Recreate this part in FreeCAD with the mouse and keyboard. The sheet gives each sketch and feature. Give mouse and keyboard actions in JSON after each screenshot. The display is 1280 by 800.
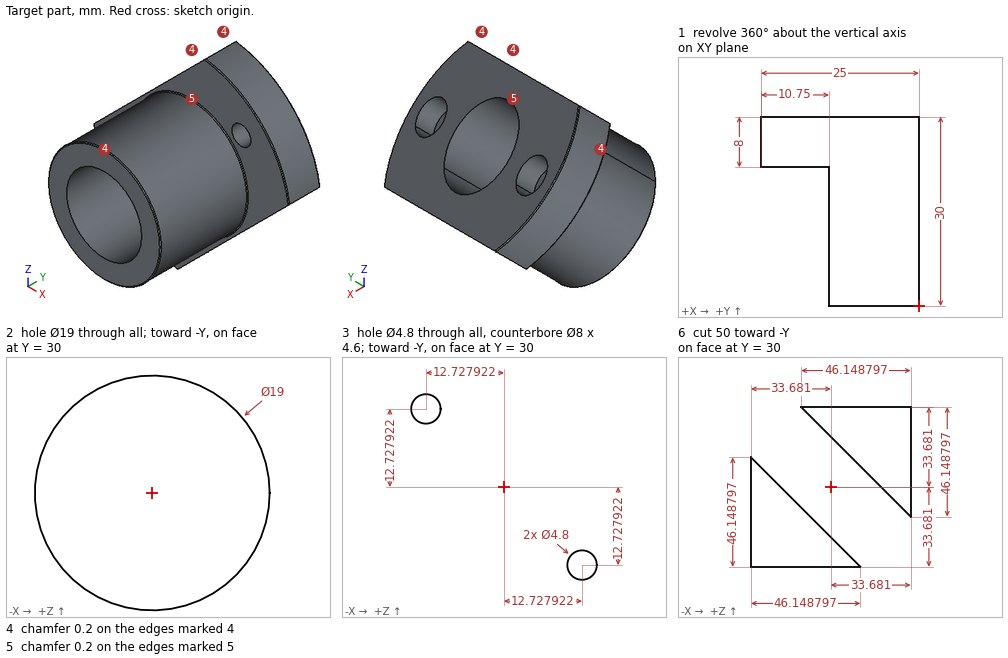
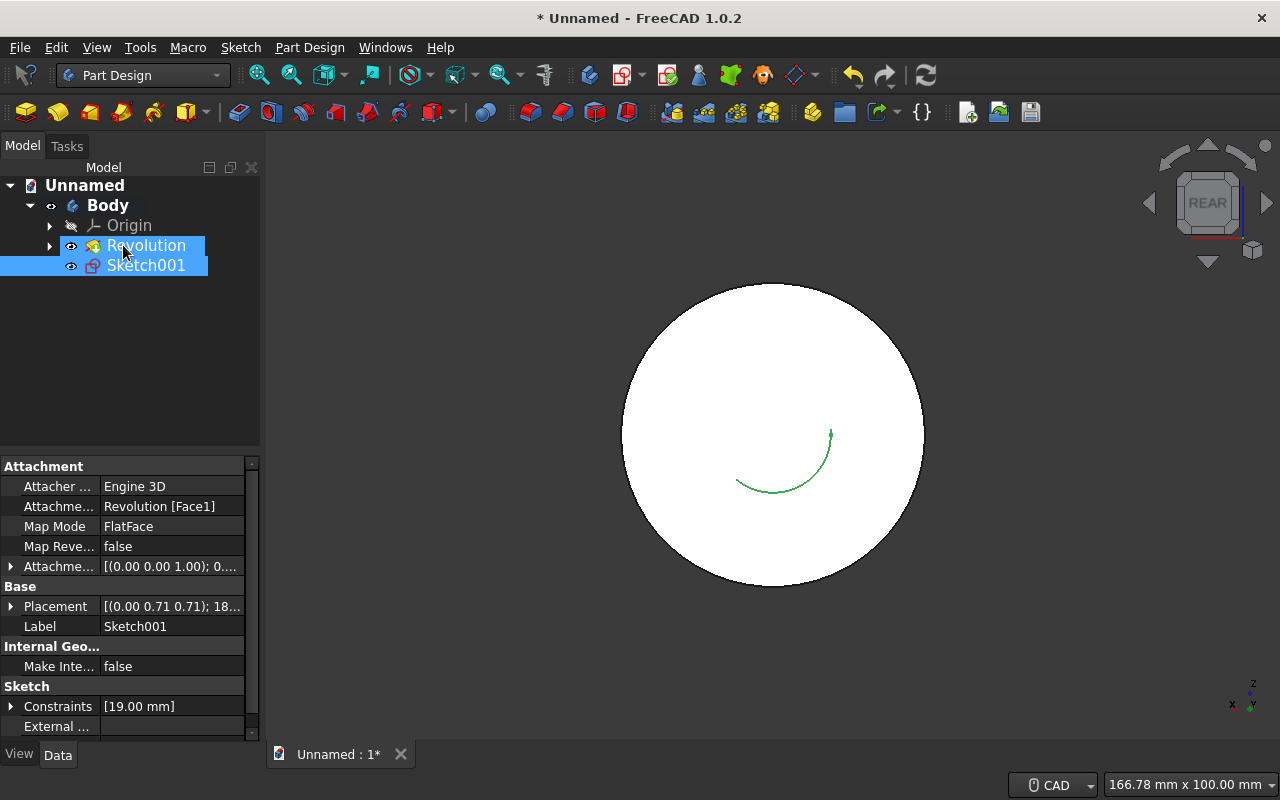
{"action": "left_click", "coordinate": [272, 112]}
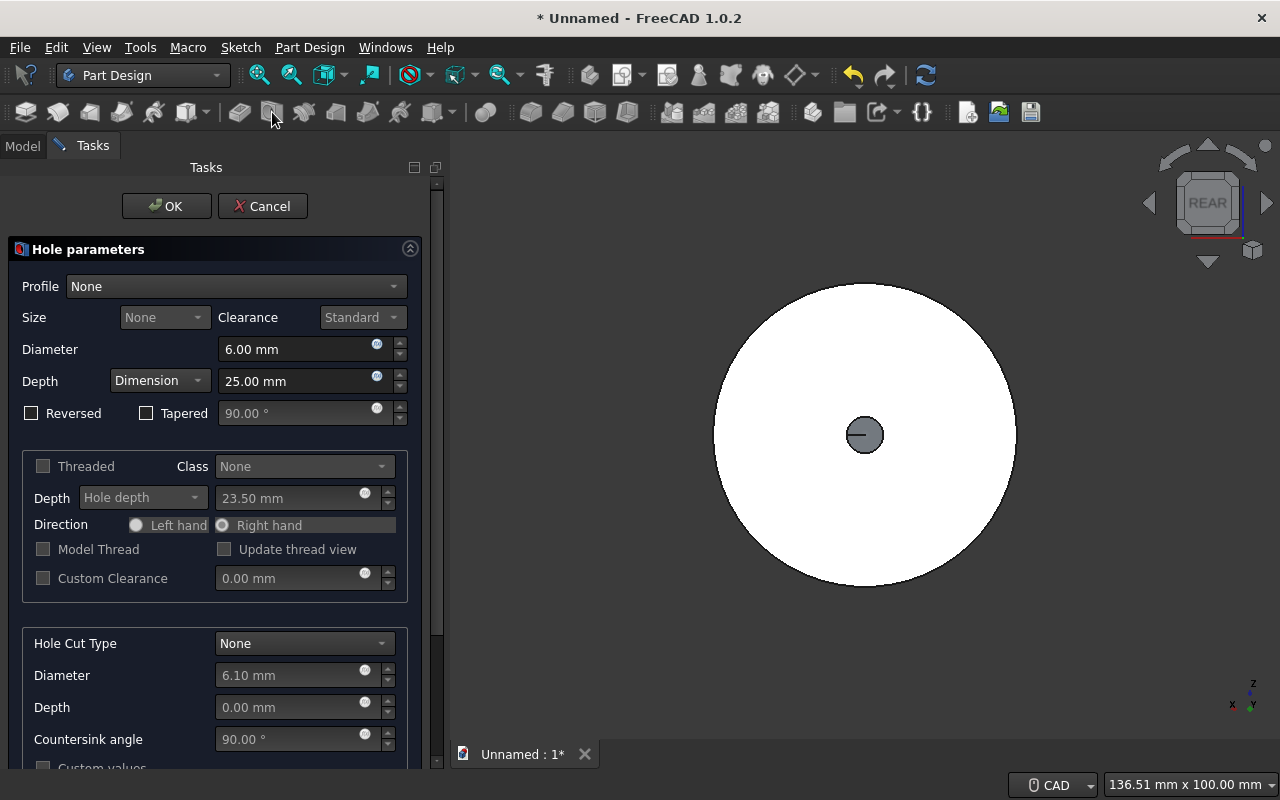
{"action": "triple_click", "coordinate": [305, 349]}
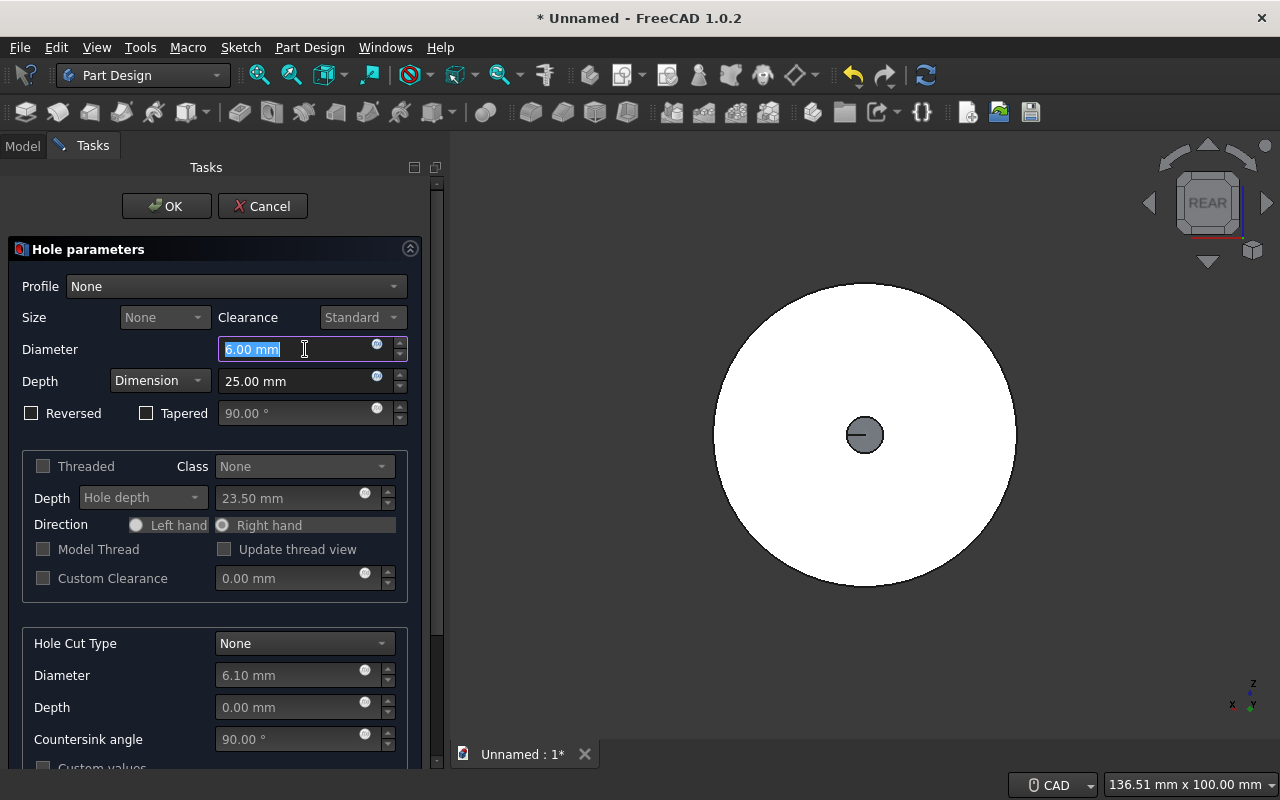
{"action": "type", "text": "19"}
{"action": "key", "text": "Tab"}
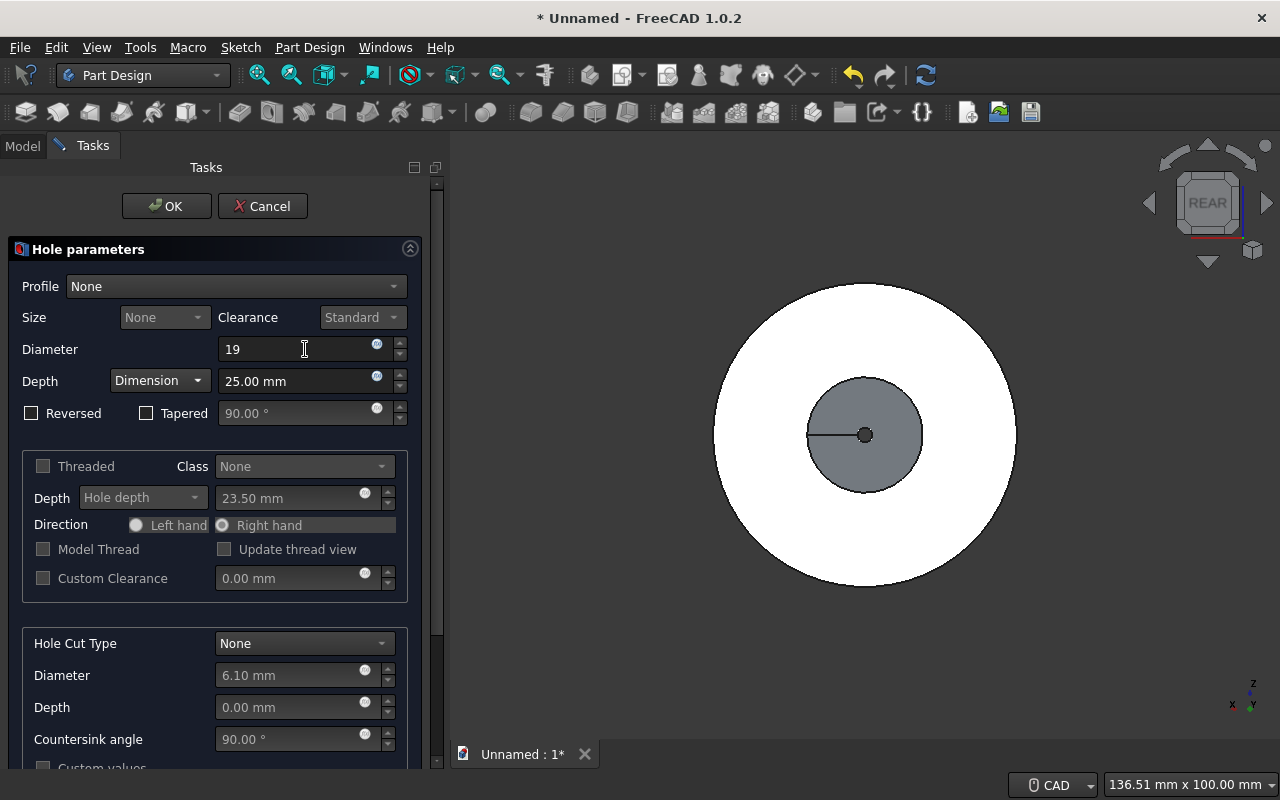
{"action": "left_click", "coordinate": [161, 380]}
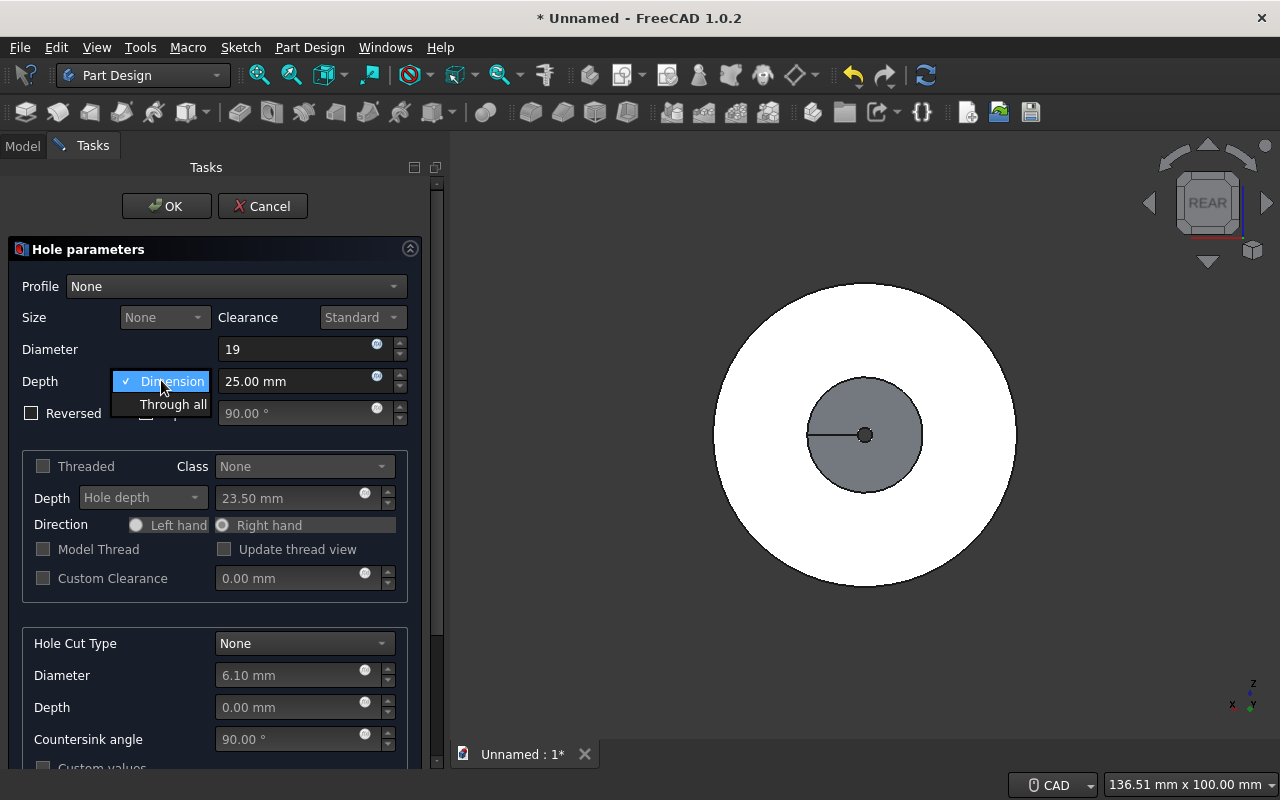
{"action": "left_click", "coordinate": [160, 404]}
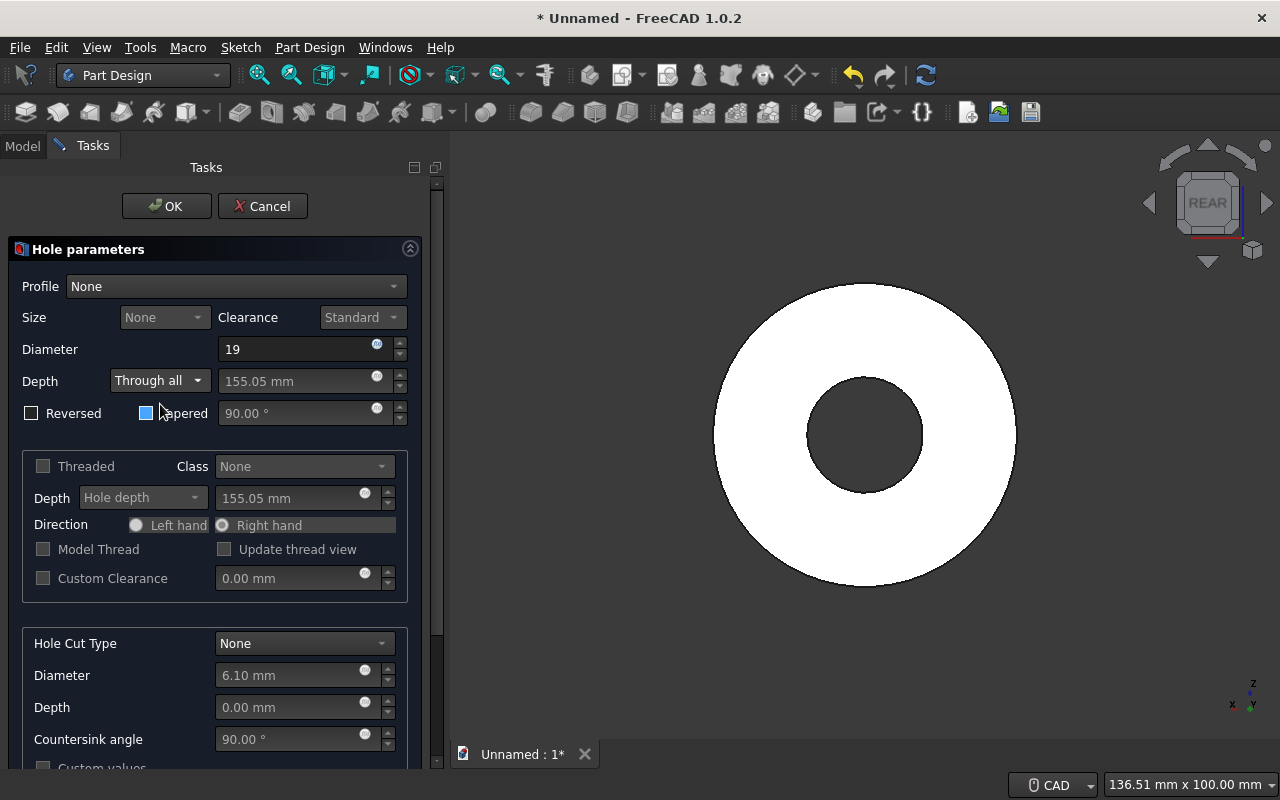
{"action": "left_click", "coordinate": [167, 206]}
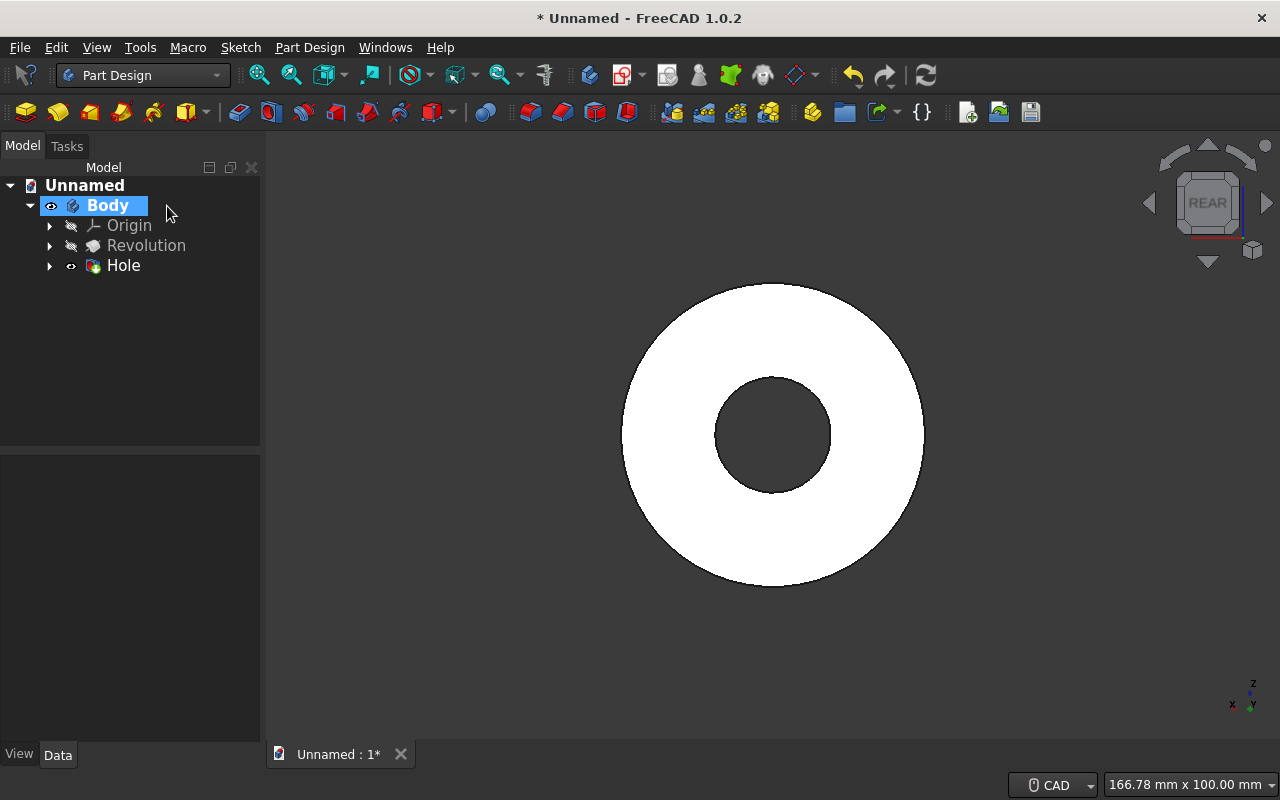
{"action": "left_click", "coordinate": [860, 391]}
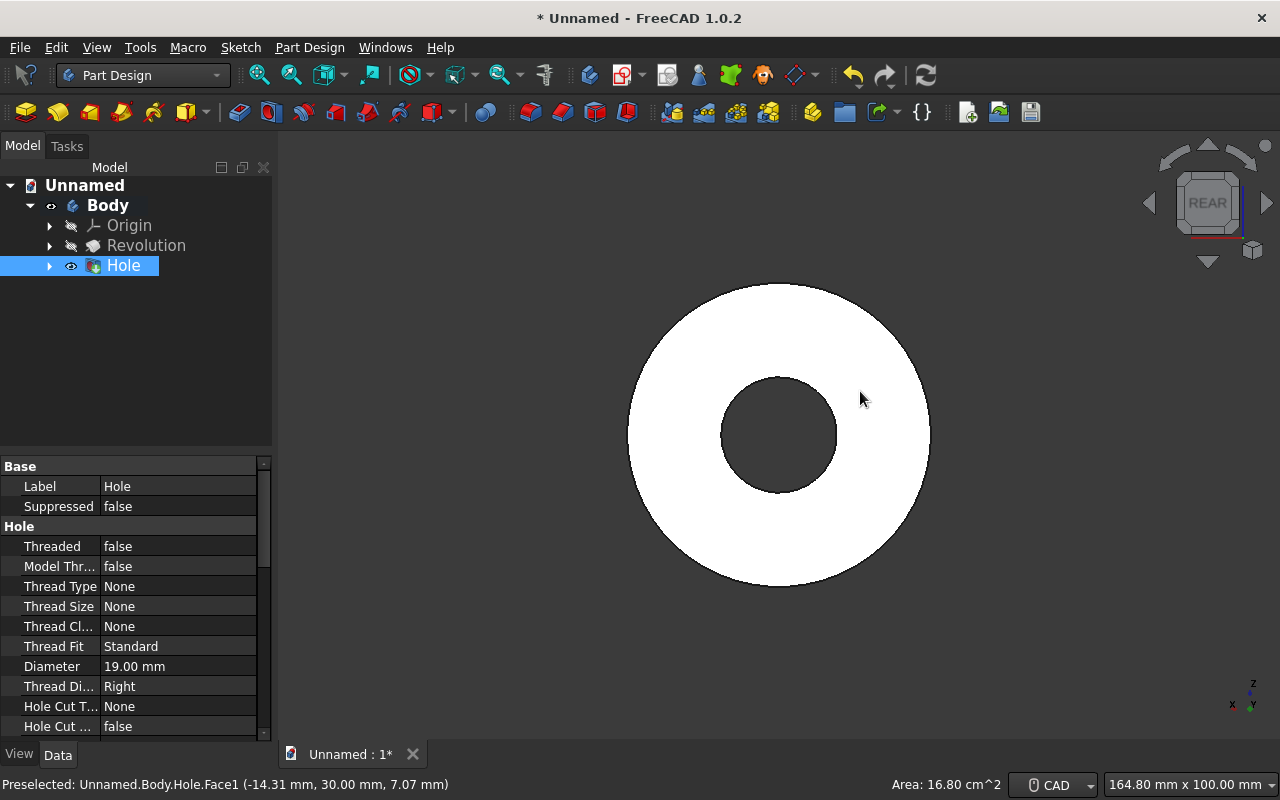
{"action": "left_click", "coordinate": [622, 76]}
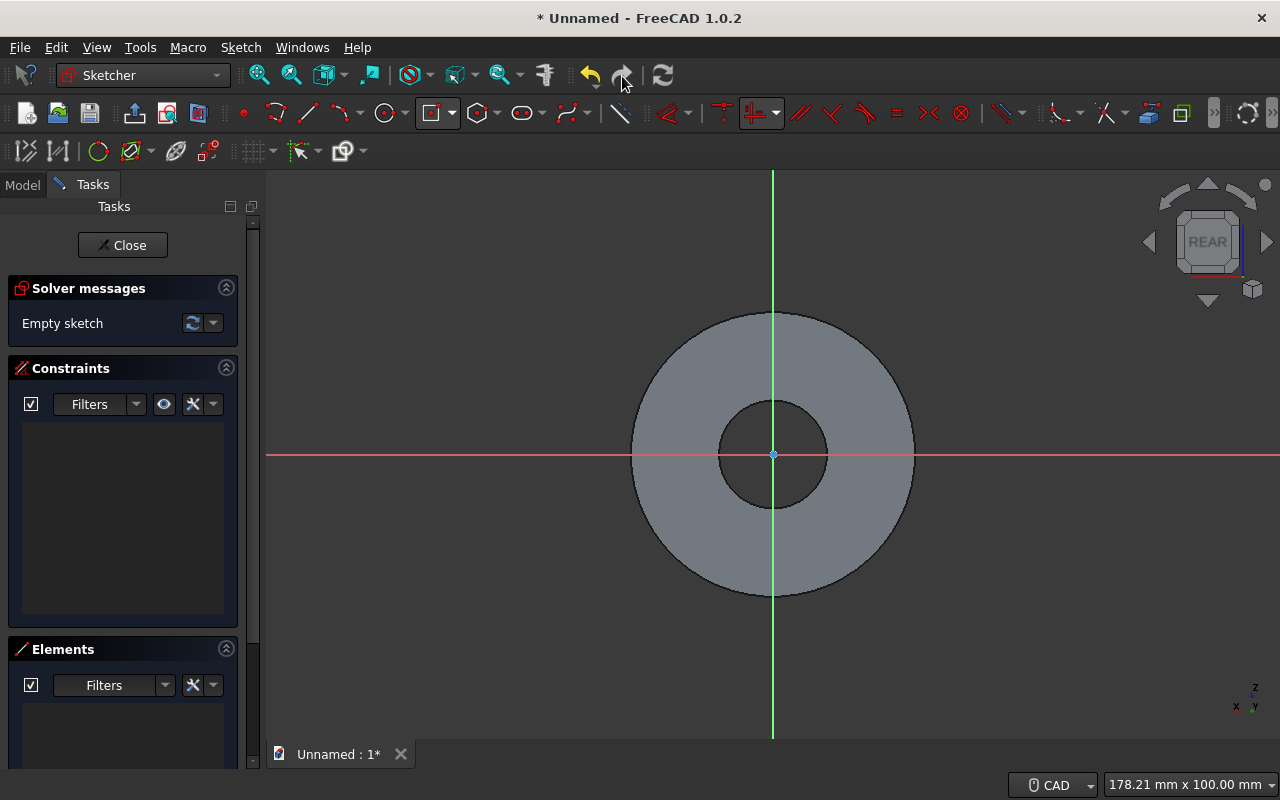
{"action": "scroll", "coordinate": [829, 455], "scroll_direction": "up", "scroll_amount": 4}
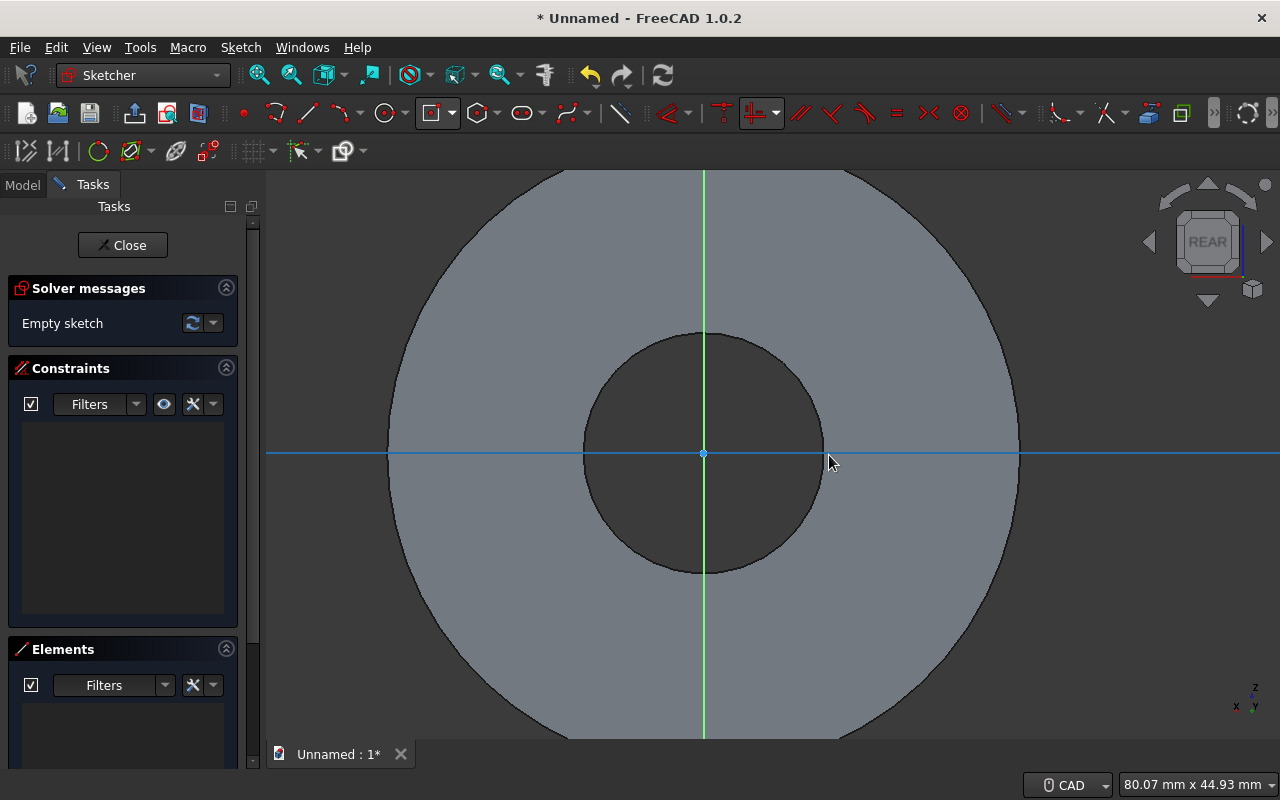
{"action": "left_click", "coordinate": [386, 114]}